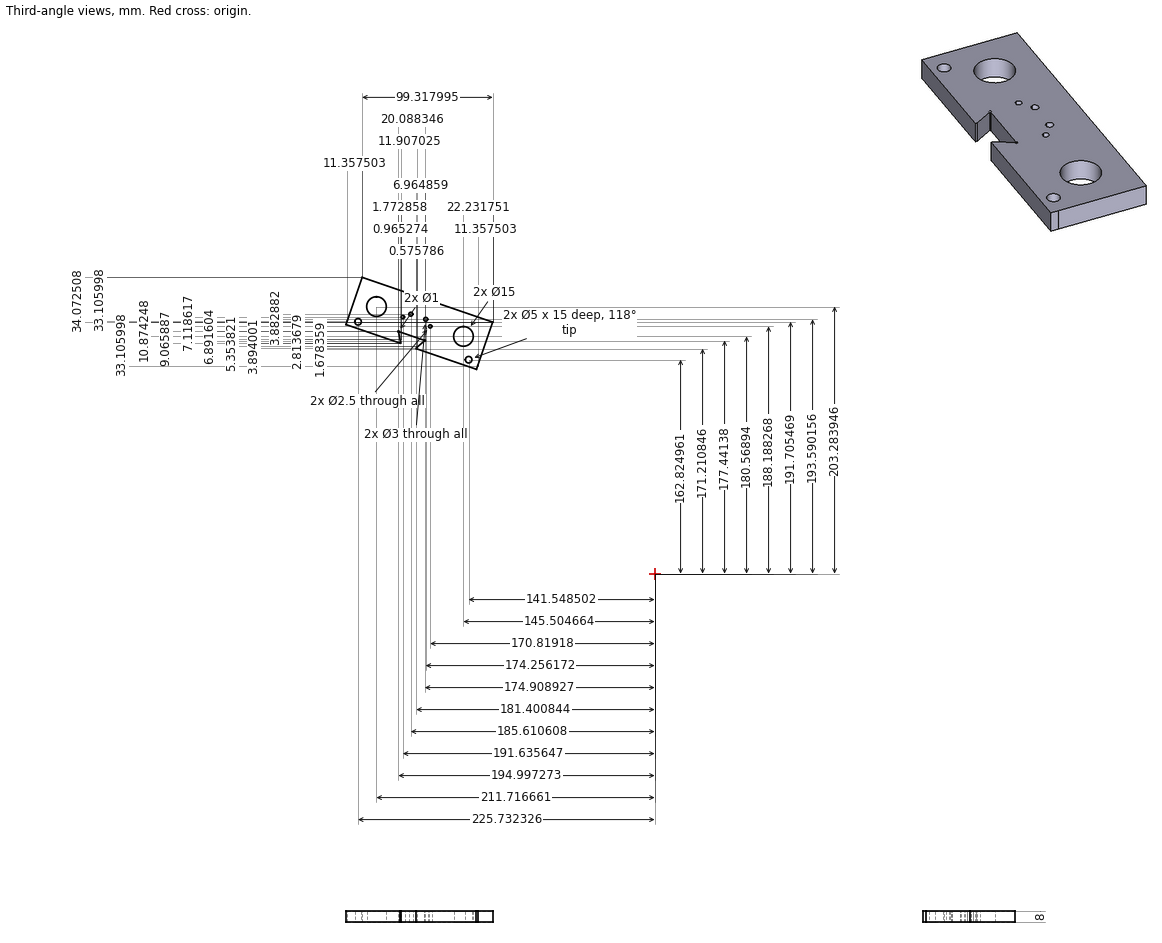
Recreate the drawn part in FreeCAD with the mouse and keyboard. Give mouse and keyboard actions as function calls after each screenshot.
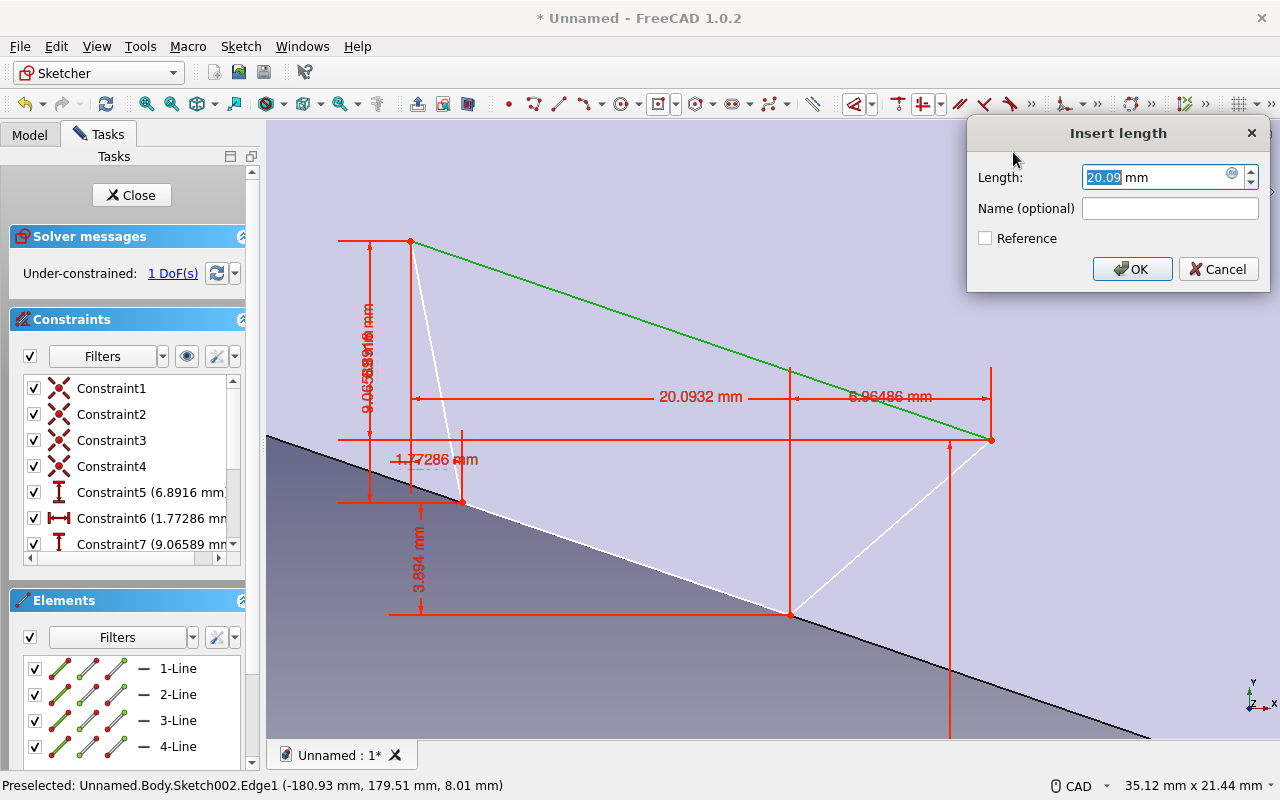
text(20.088346)
key(Return)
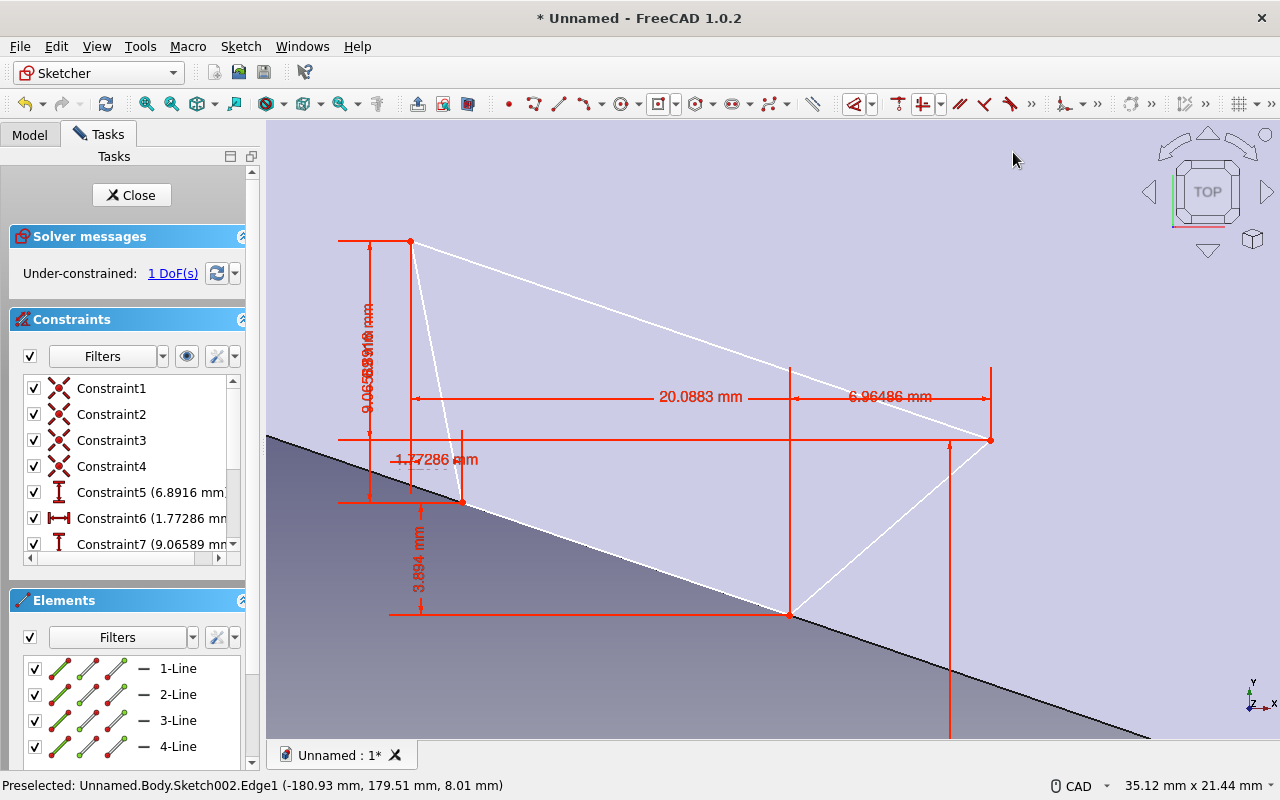
click(991, 440)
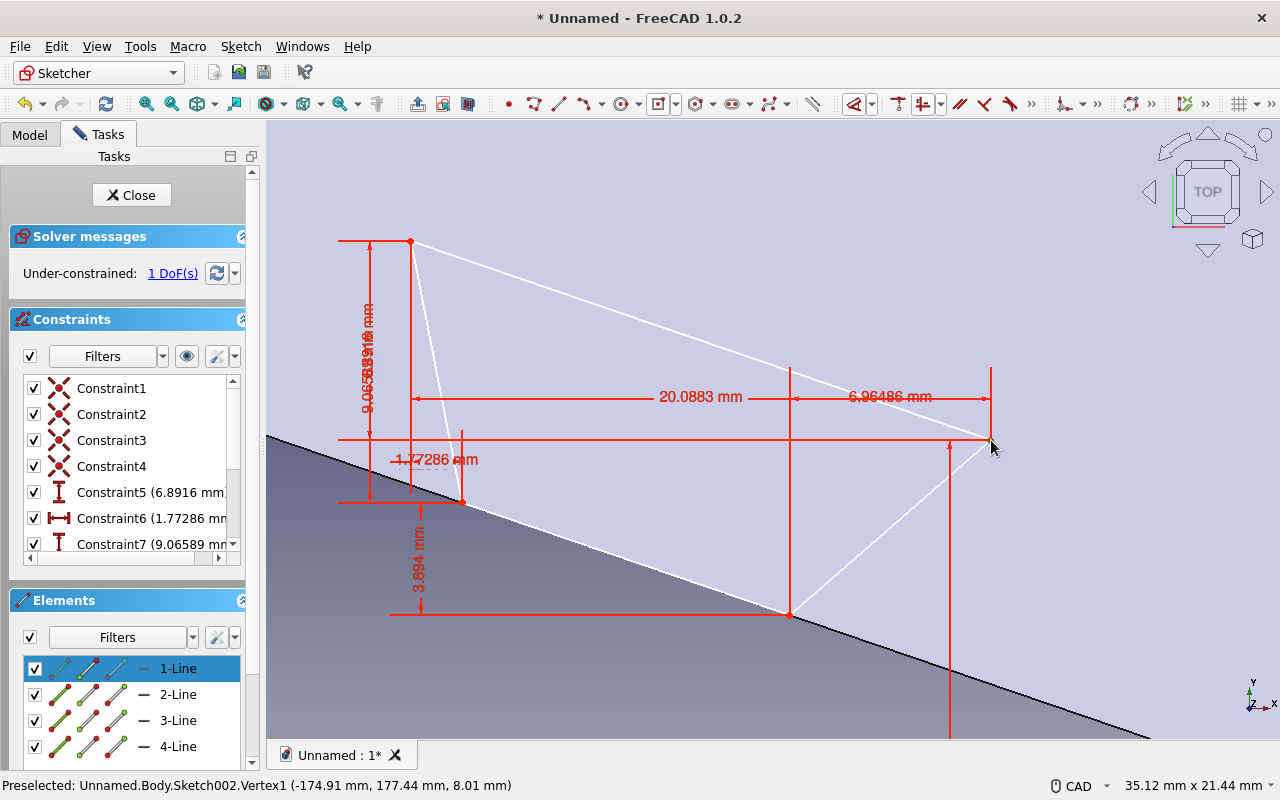
click(872, 104)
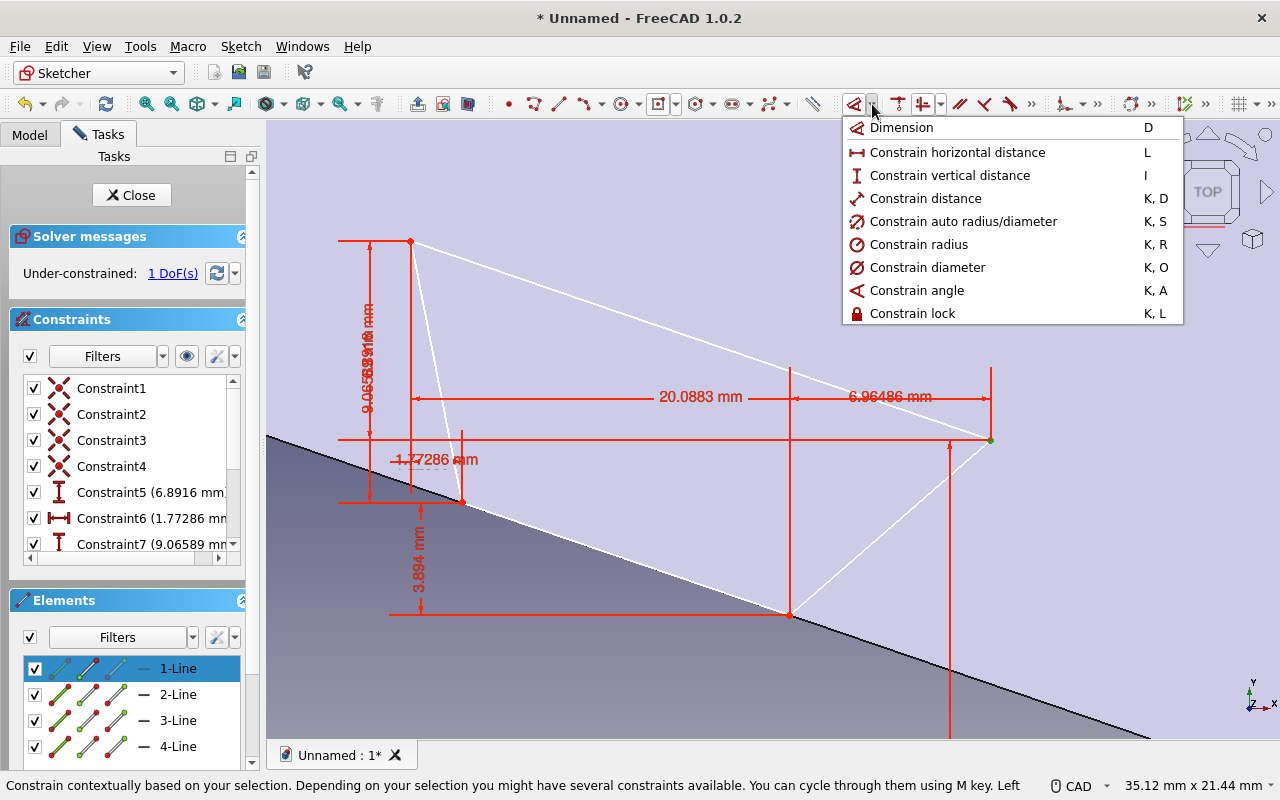
click(1013, 152)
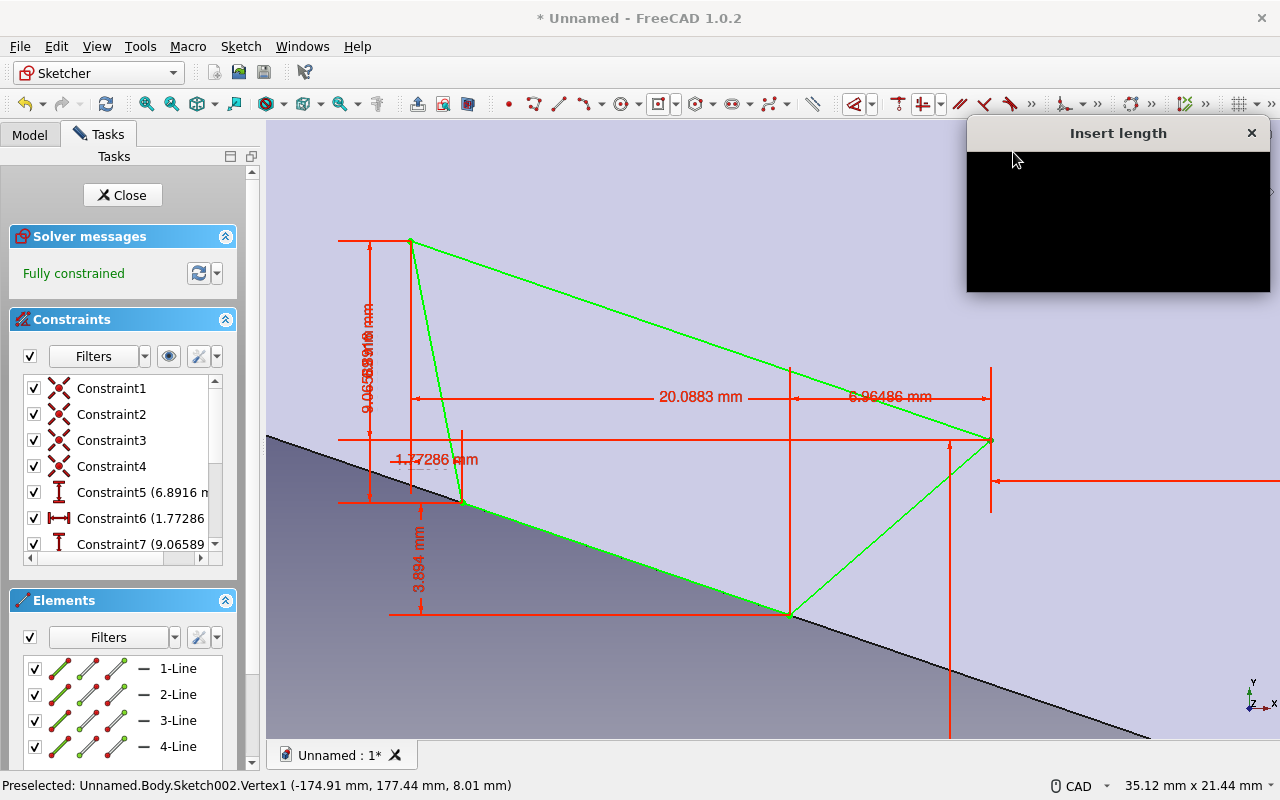
text(-174.908927)
key(Return)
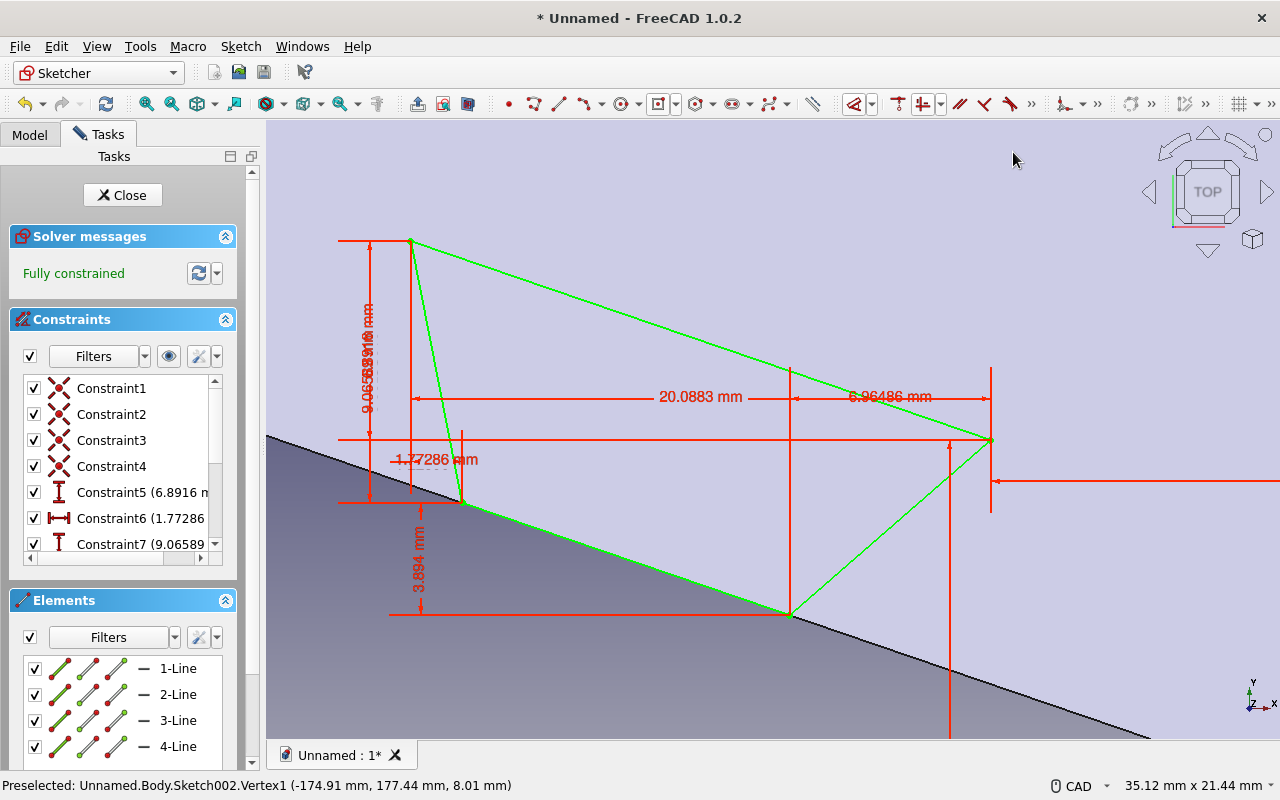
click(123, 195)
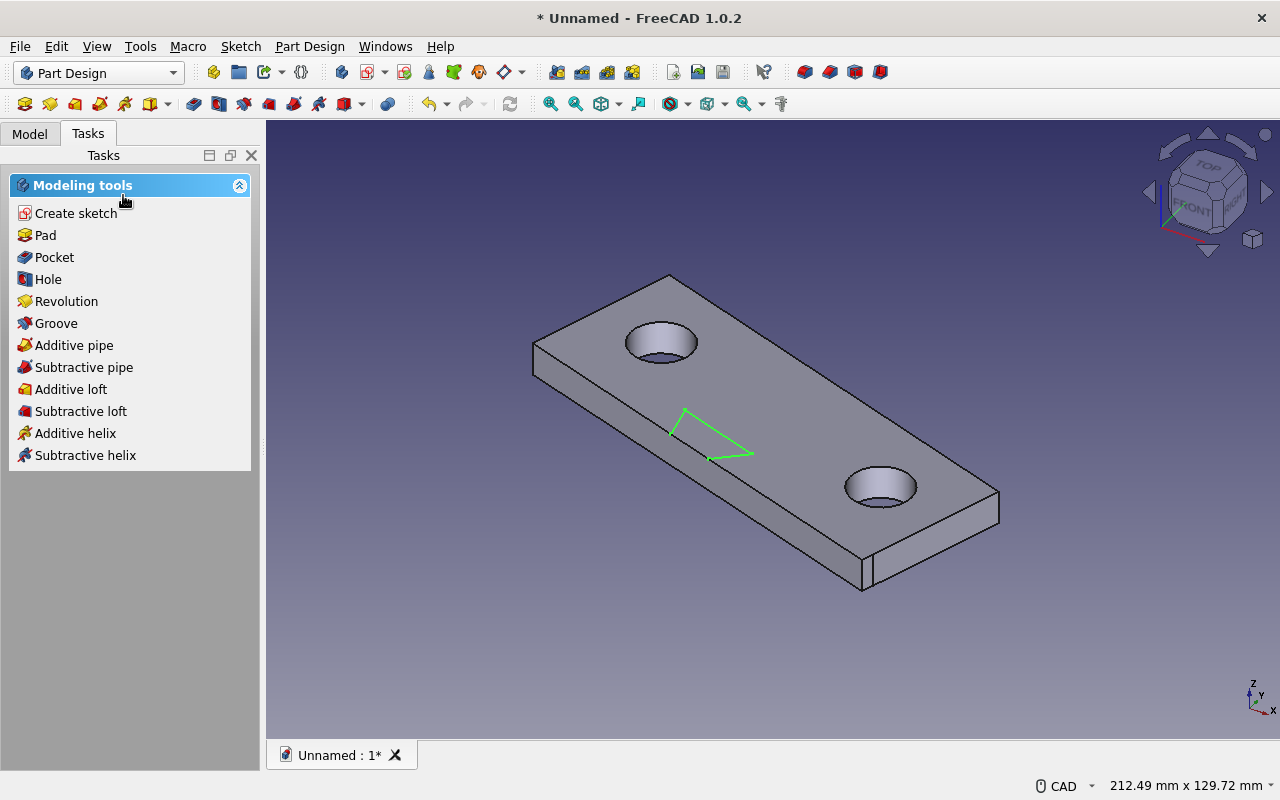
click(194, 104)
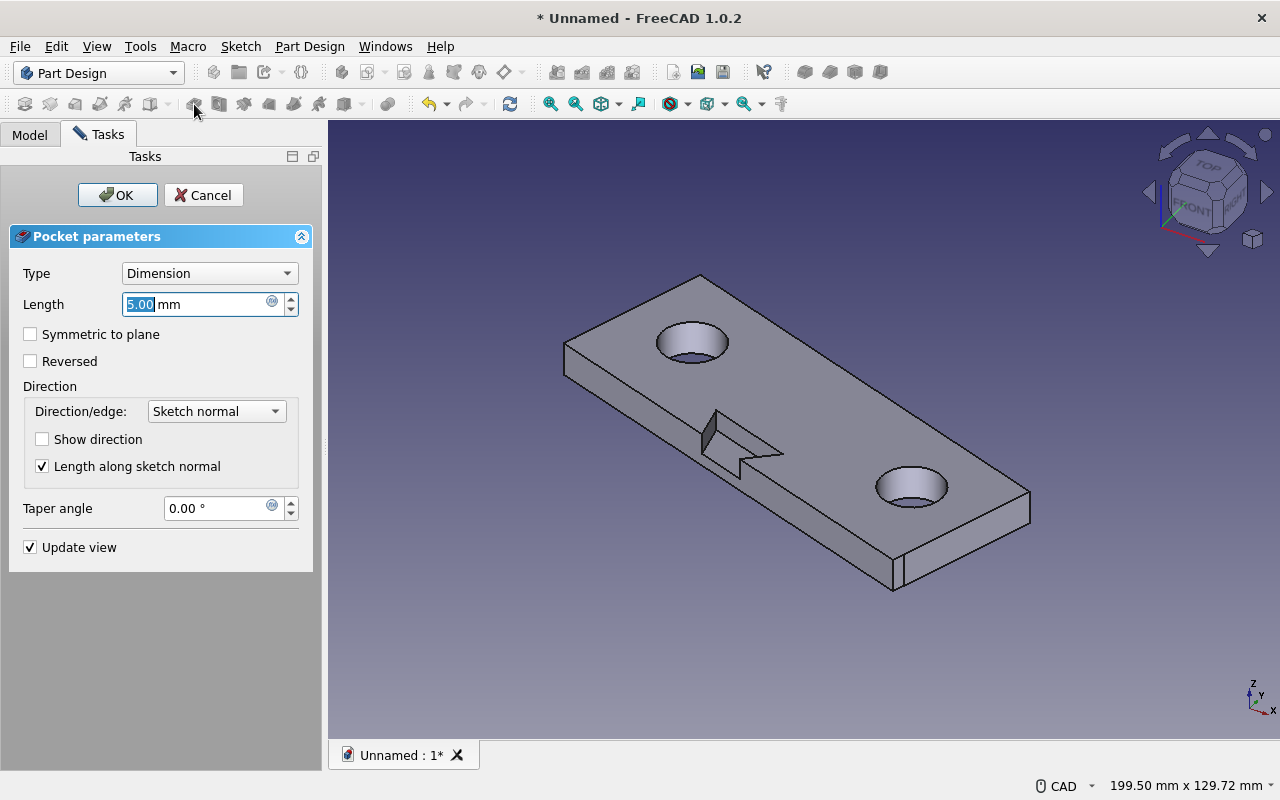
click(210, 274)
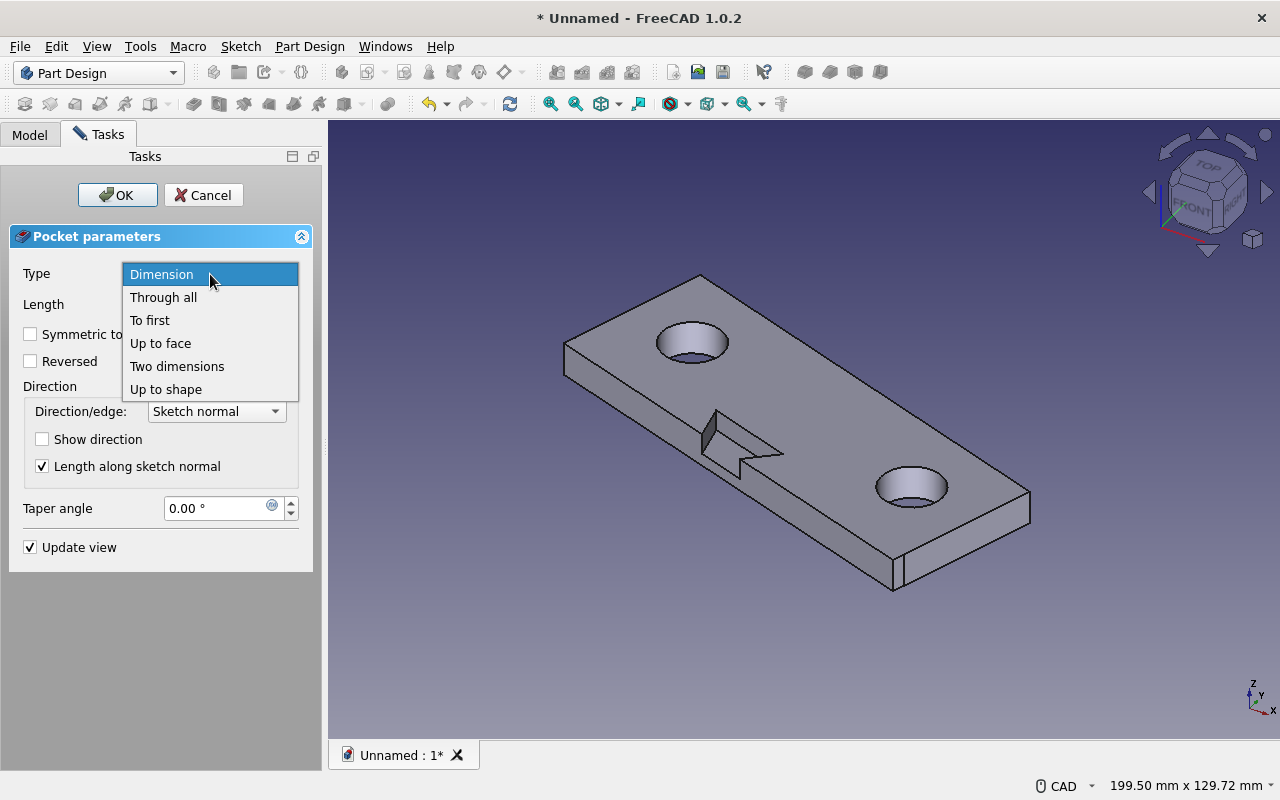
click(208, 298)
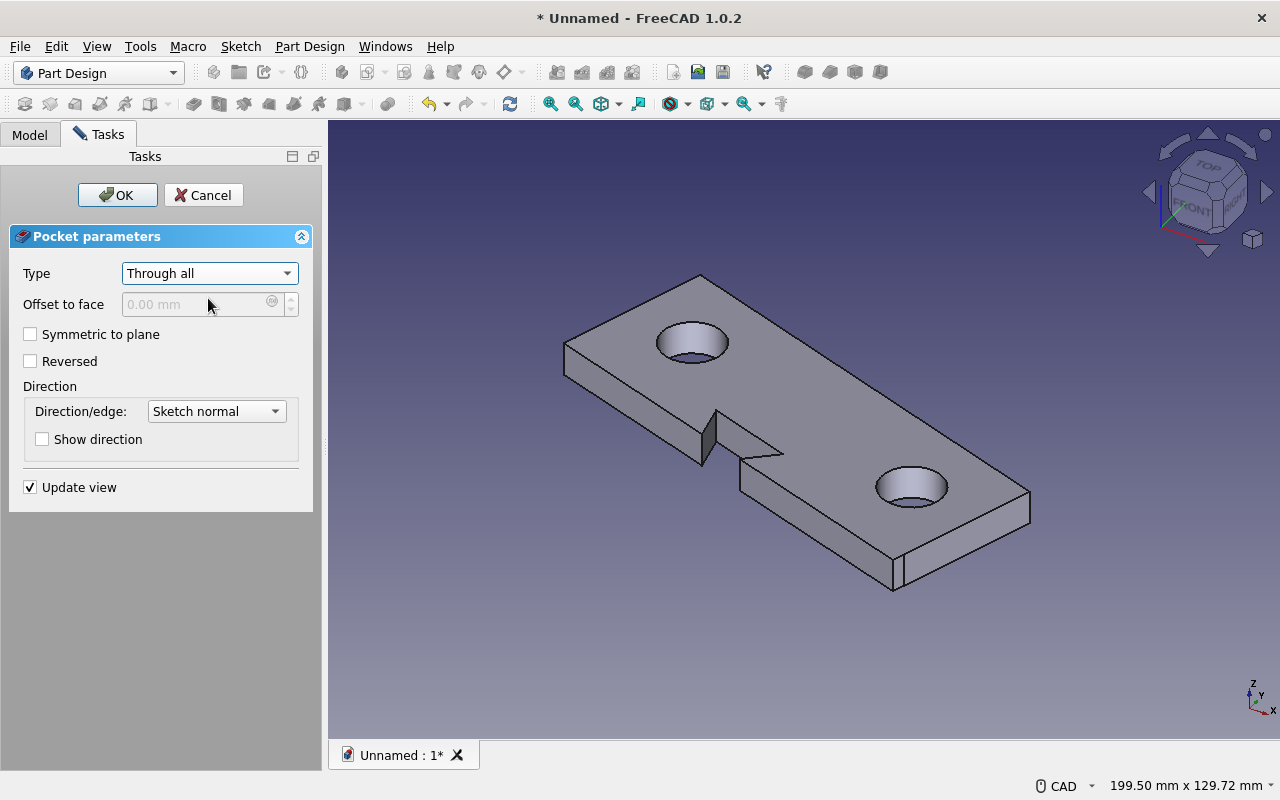
click(118, 195)